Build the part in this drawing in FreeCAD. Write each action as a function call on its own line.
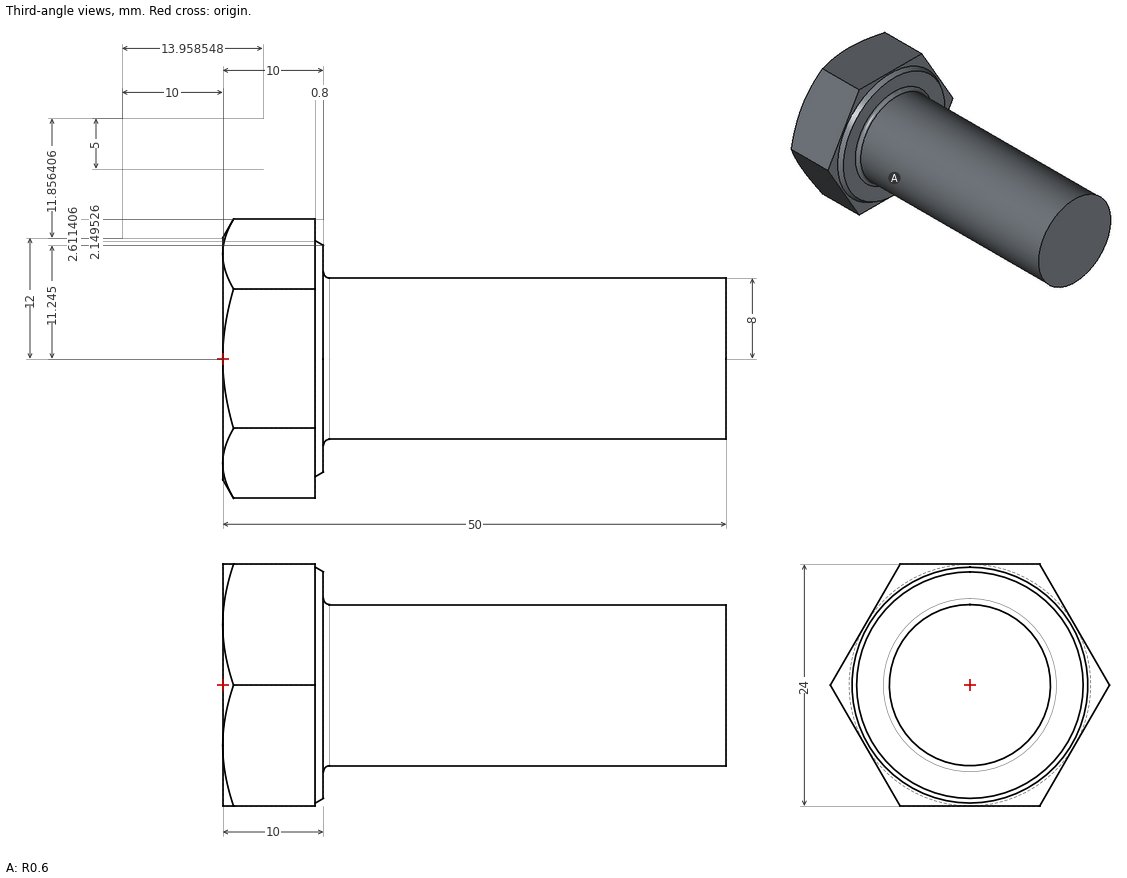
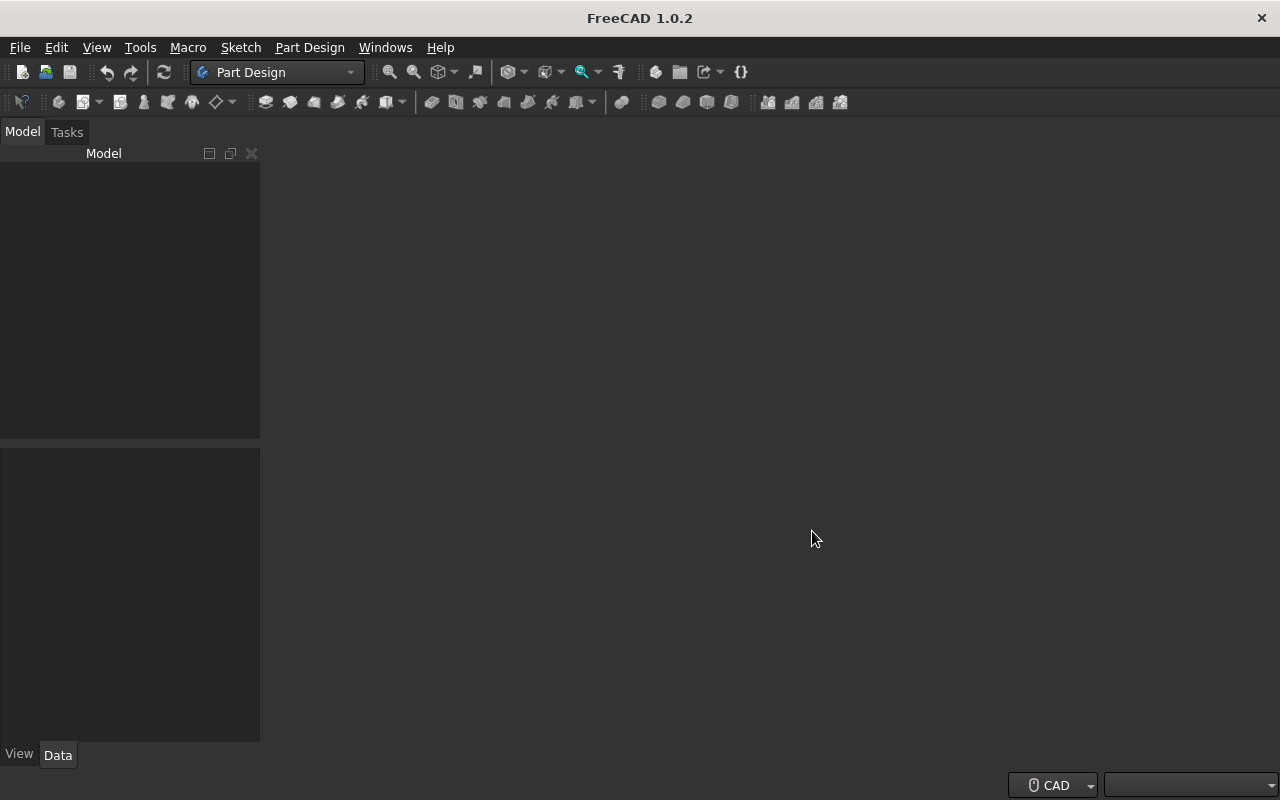
click(22, 72)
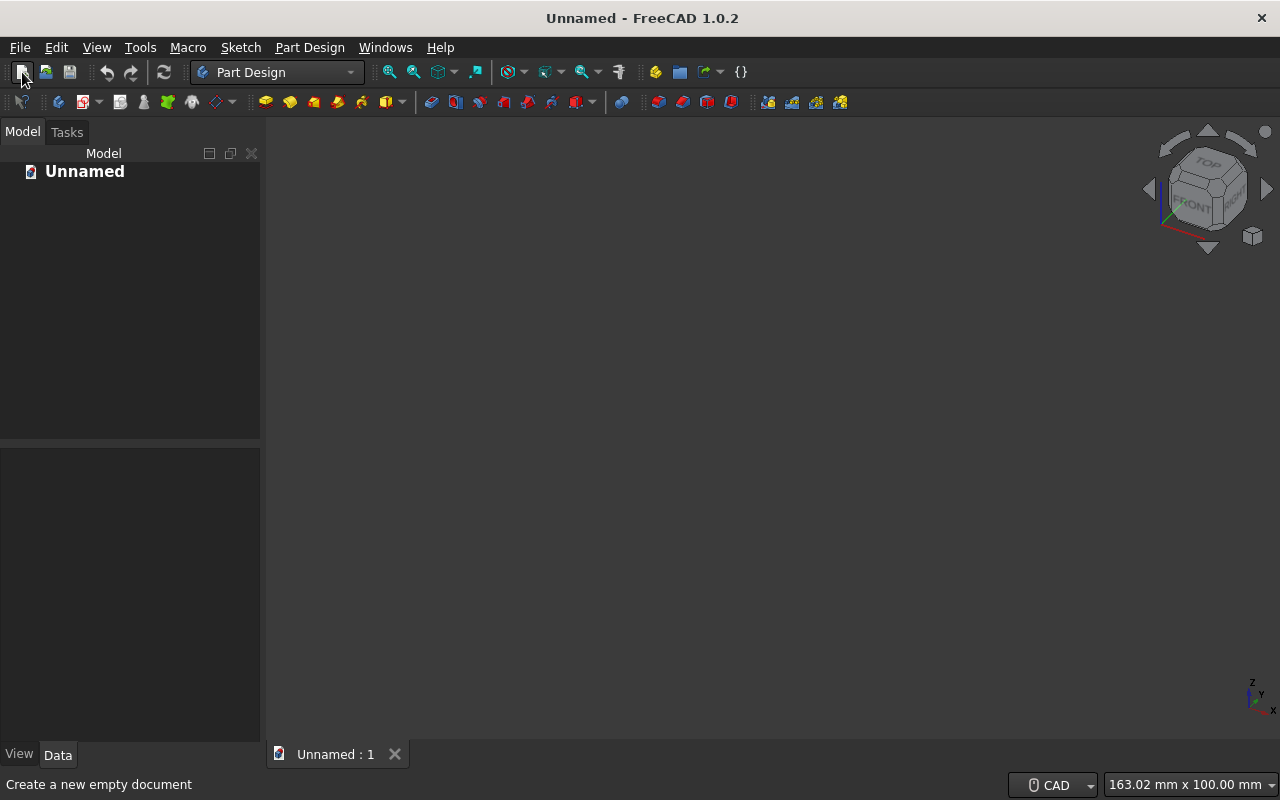
click(84, 102)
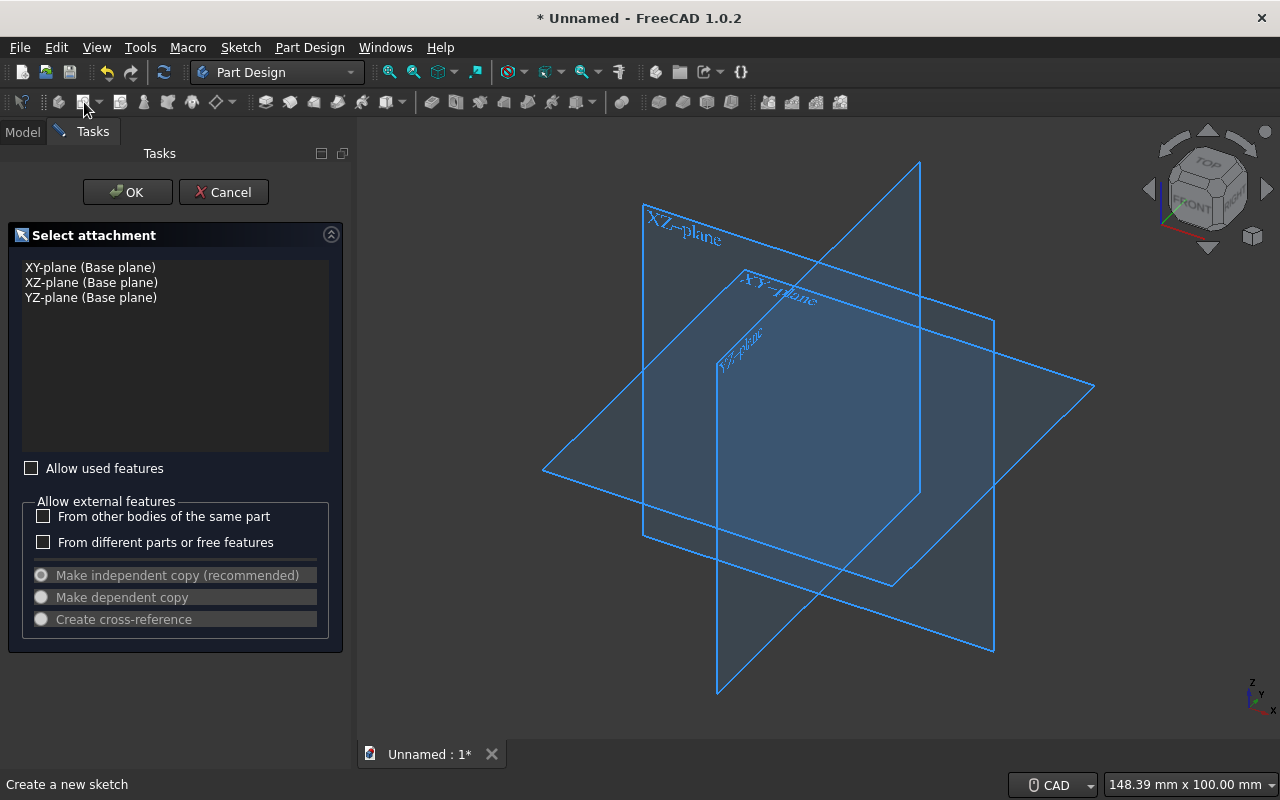
click(82, 298)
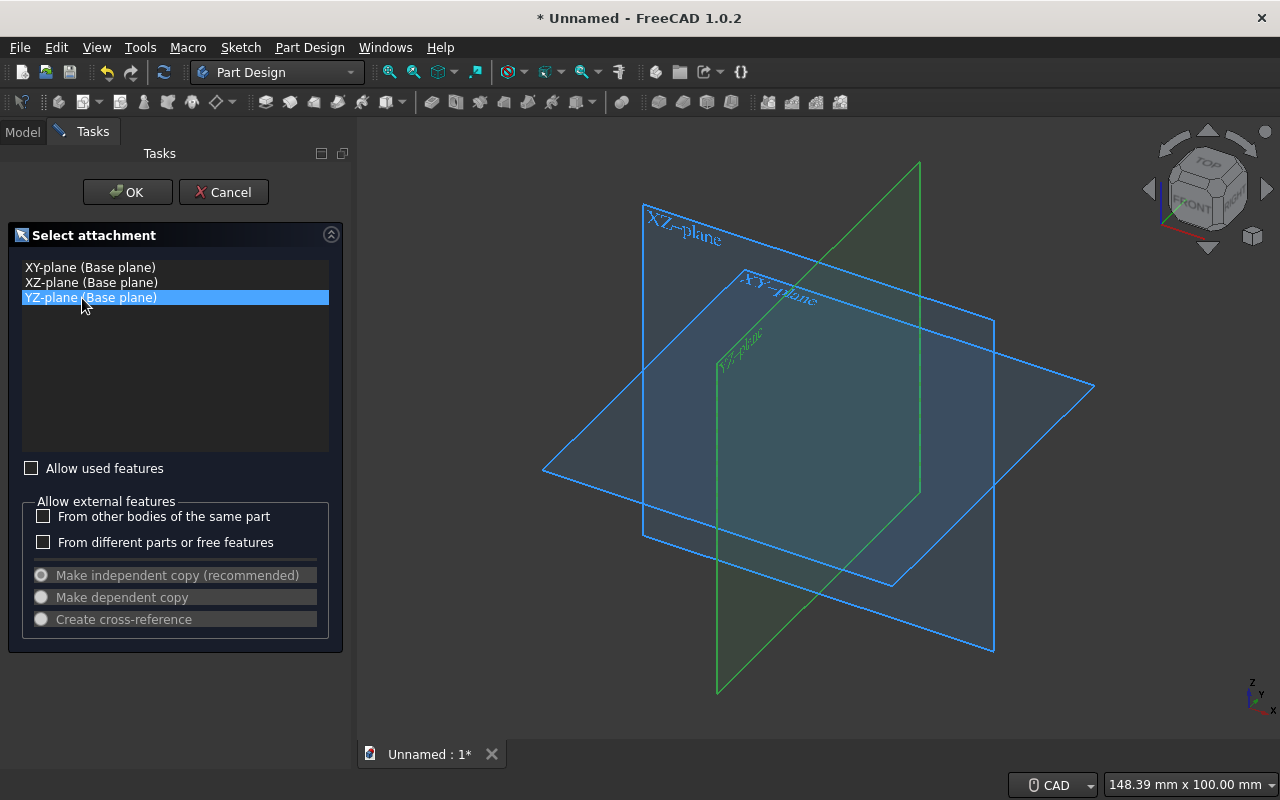
click(128, 192)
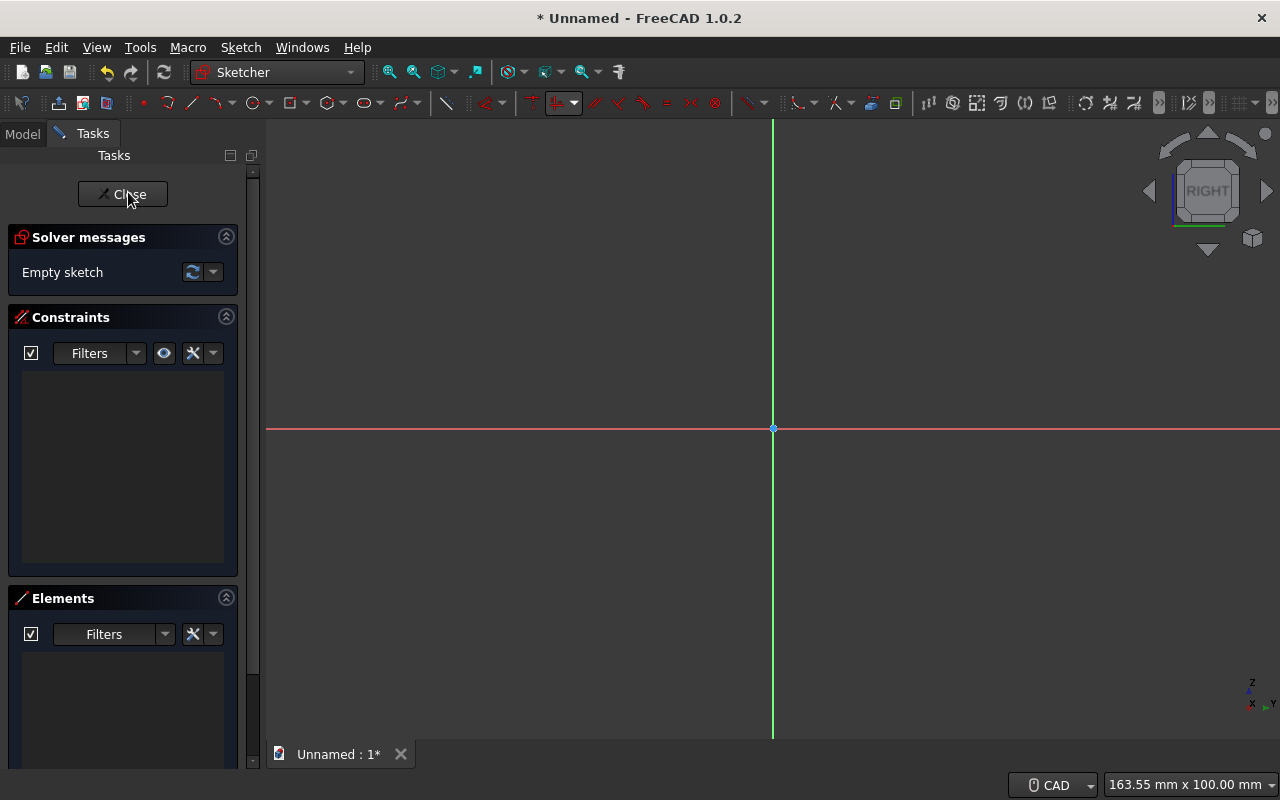
scroll(813, 429, up, 5)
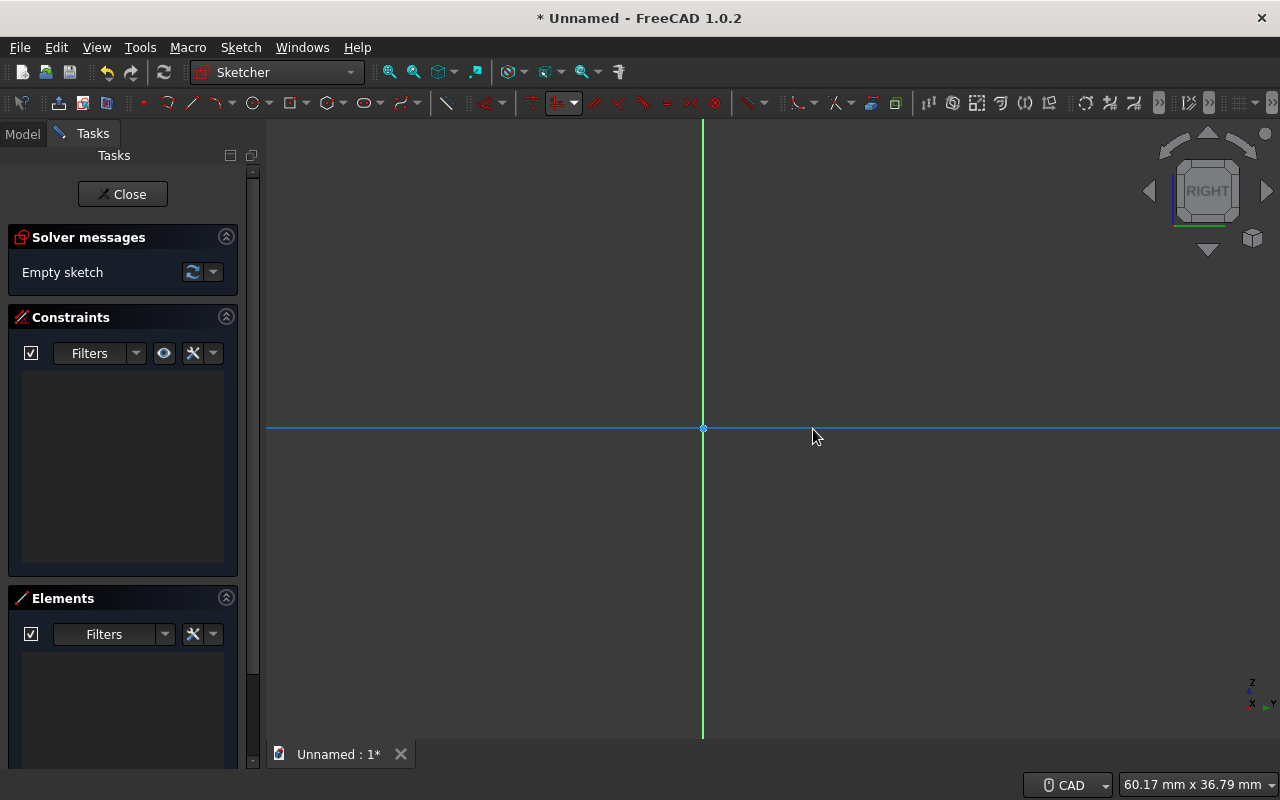
click(328, 104)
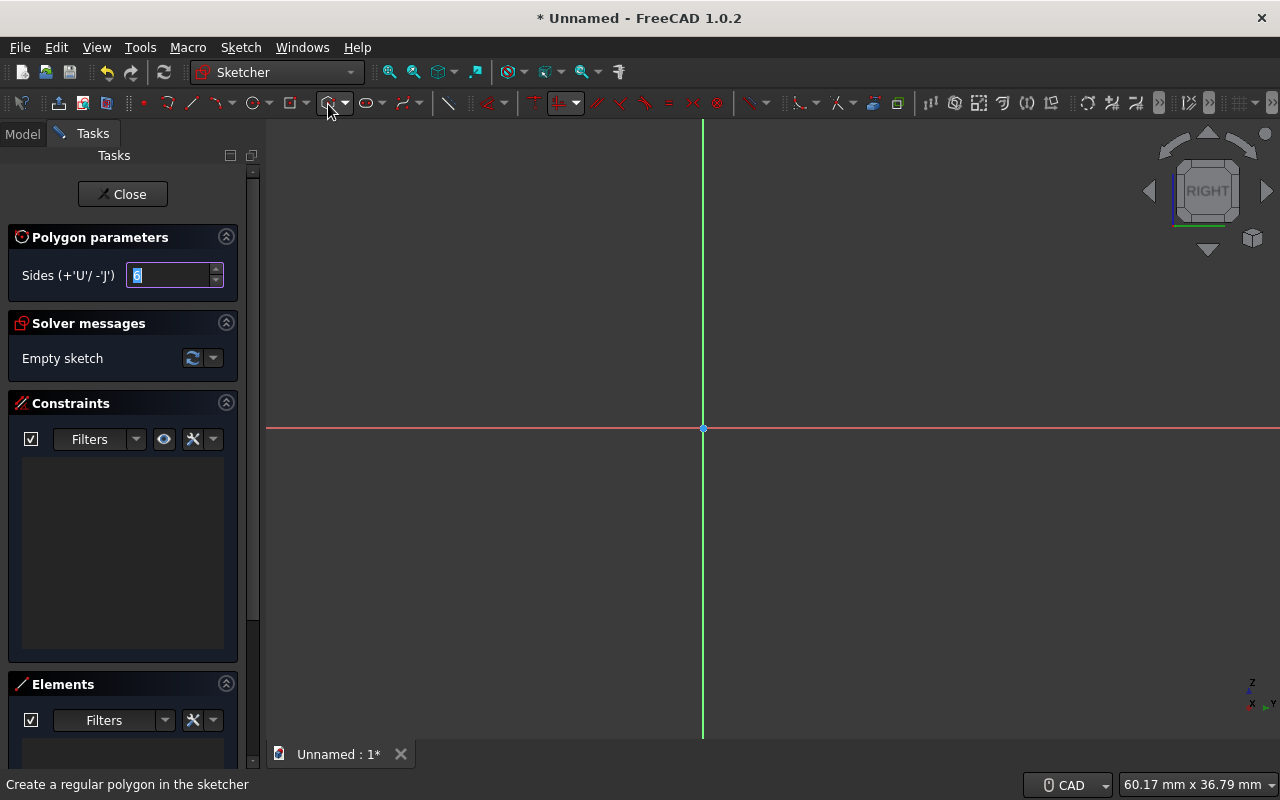
click(703, 428)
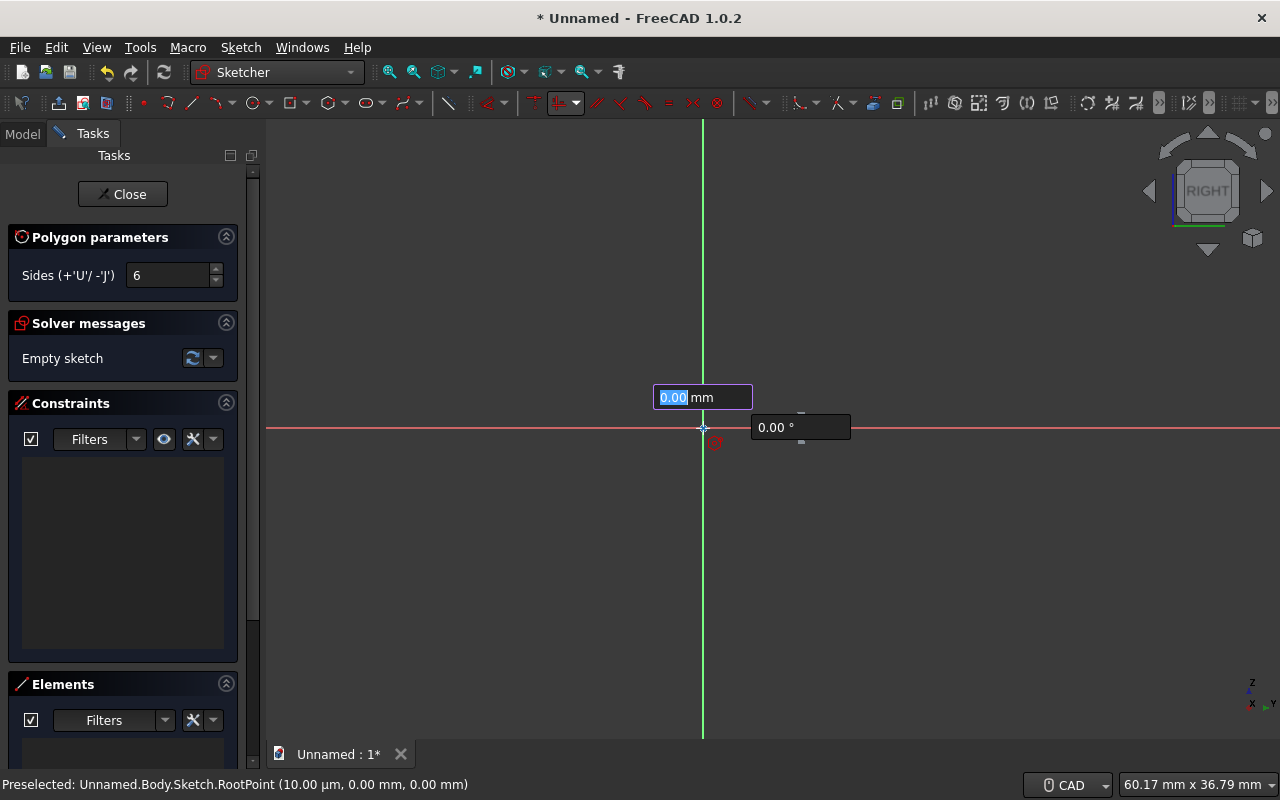
click(937, 428)
right_click(937, 428)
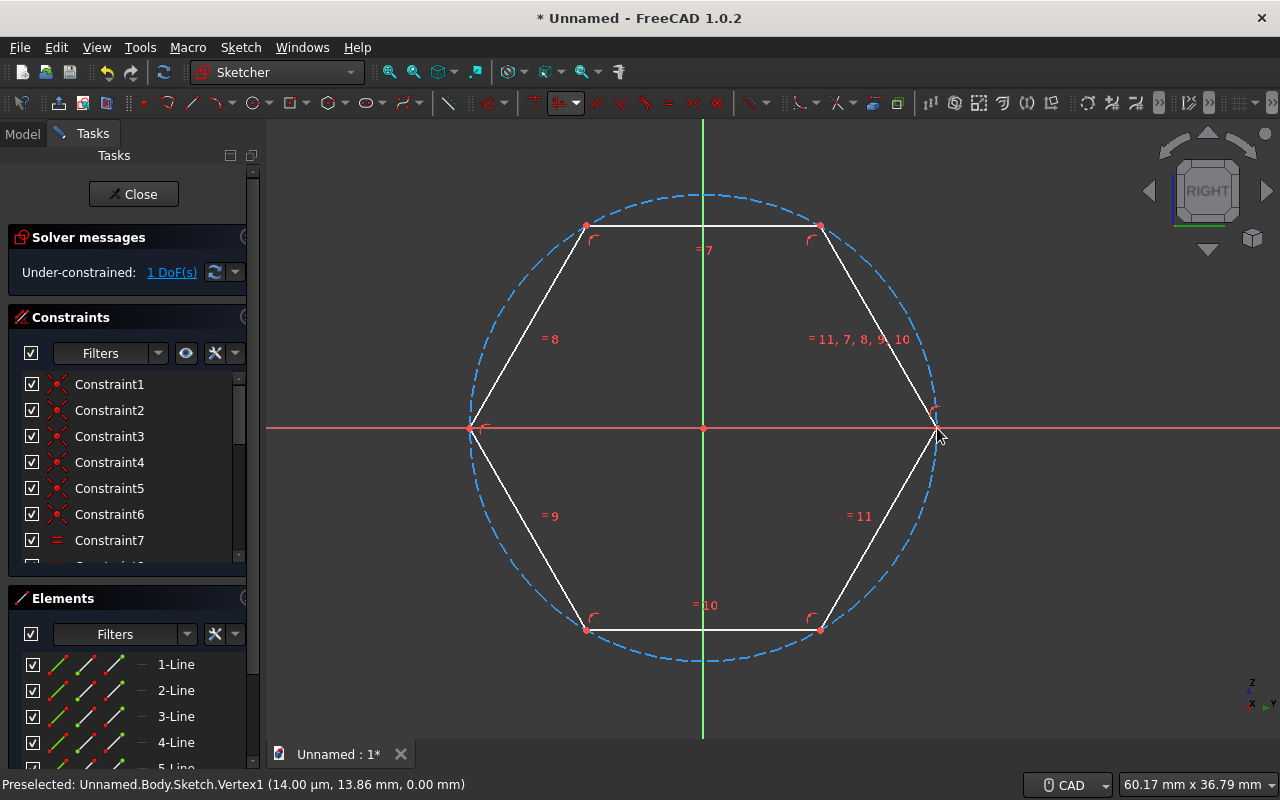
click(488, 104)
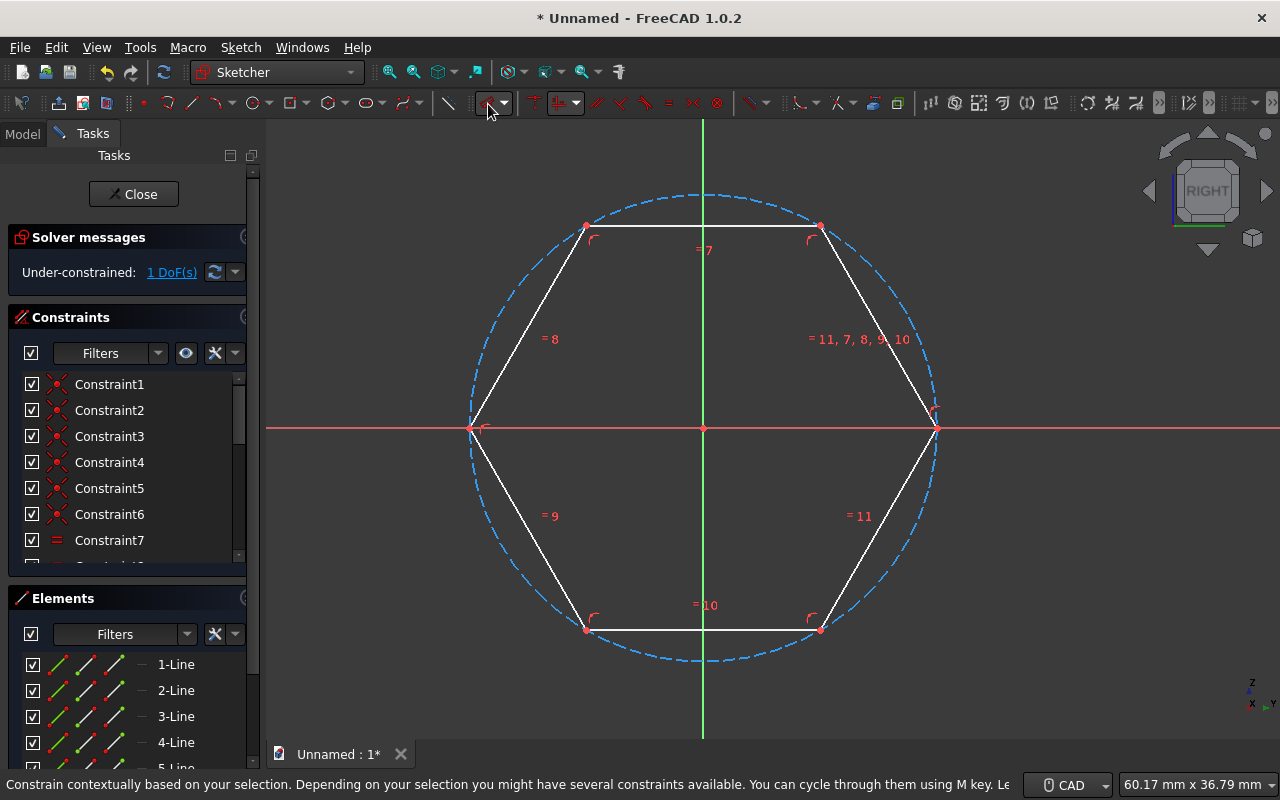
click(587, 630)